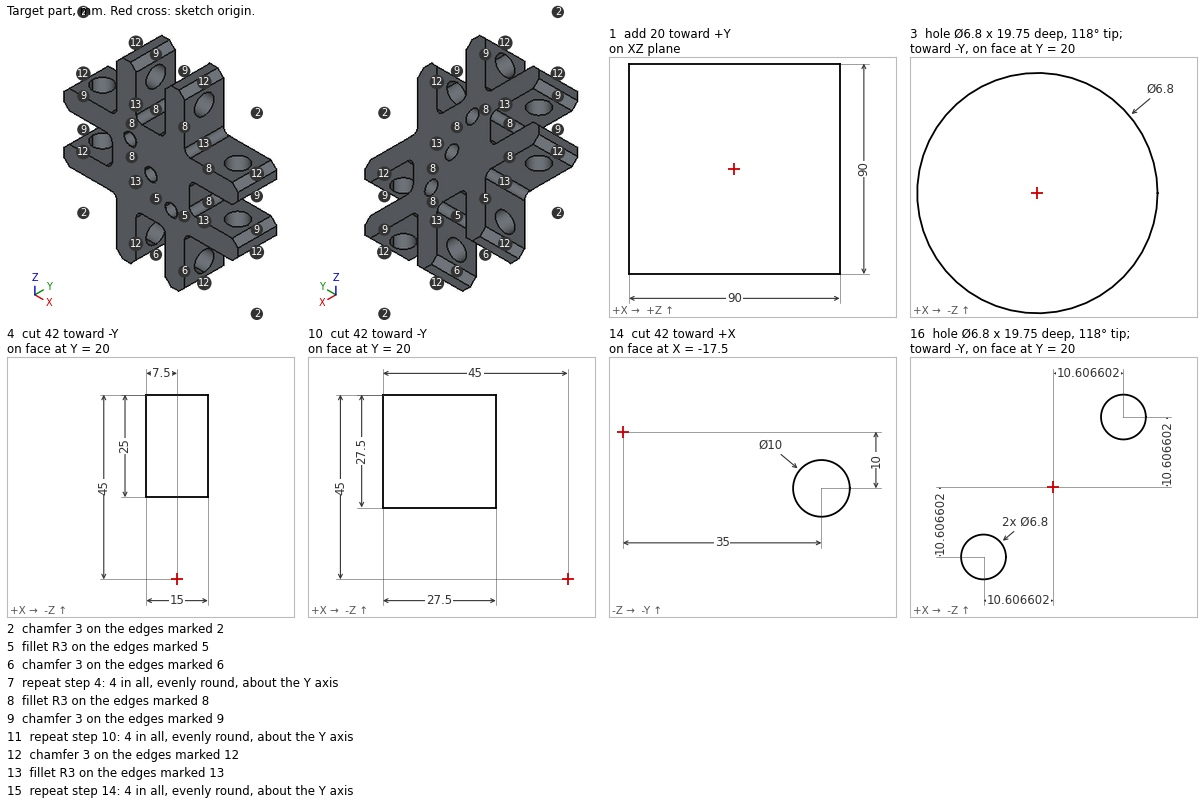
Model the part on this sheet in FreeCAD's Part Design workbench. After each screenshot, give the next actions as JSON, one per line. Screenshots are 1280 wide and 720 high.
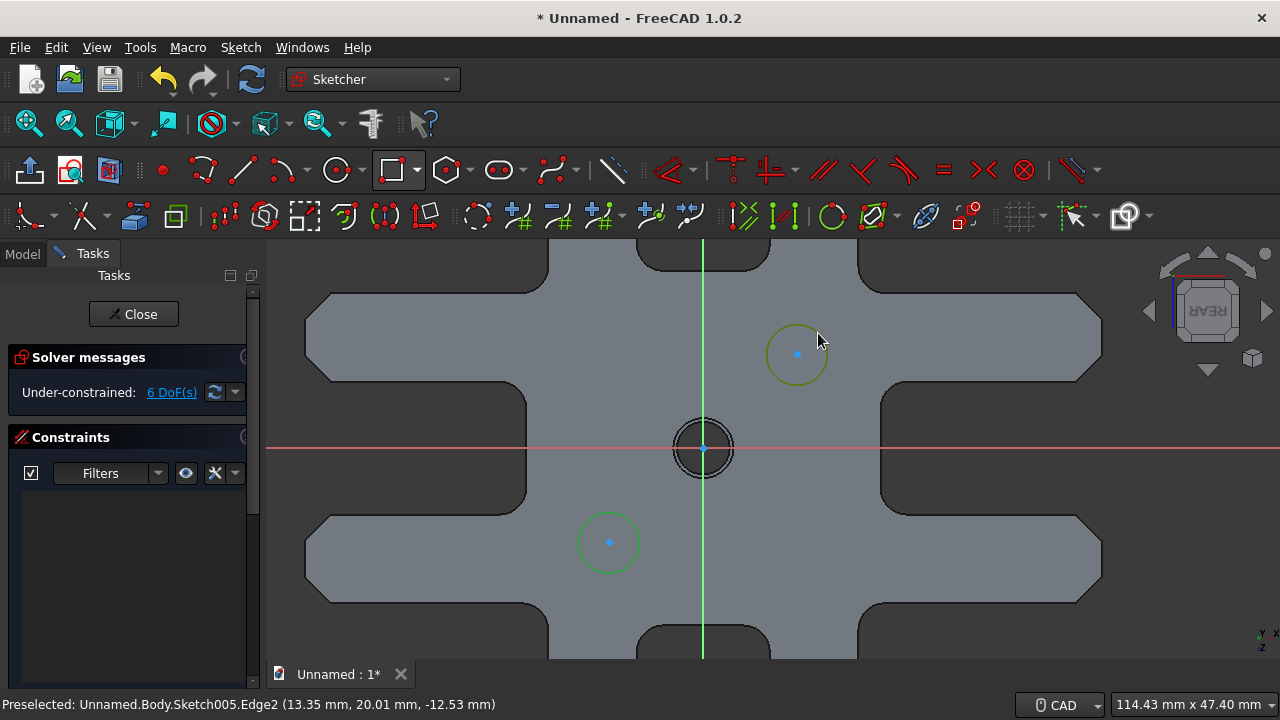
{"action": "left_click", "coordinate": [944, 170]}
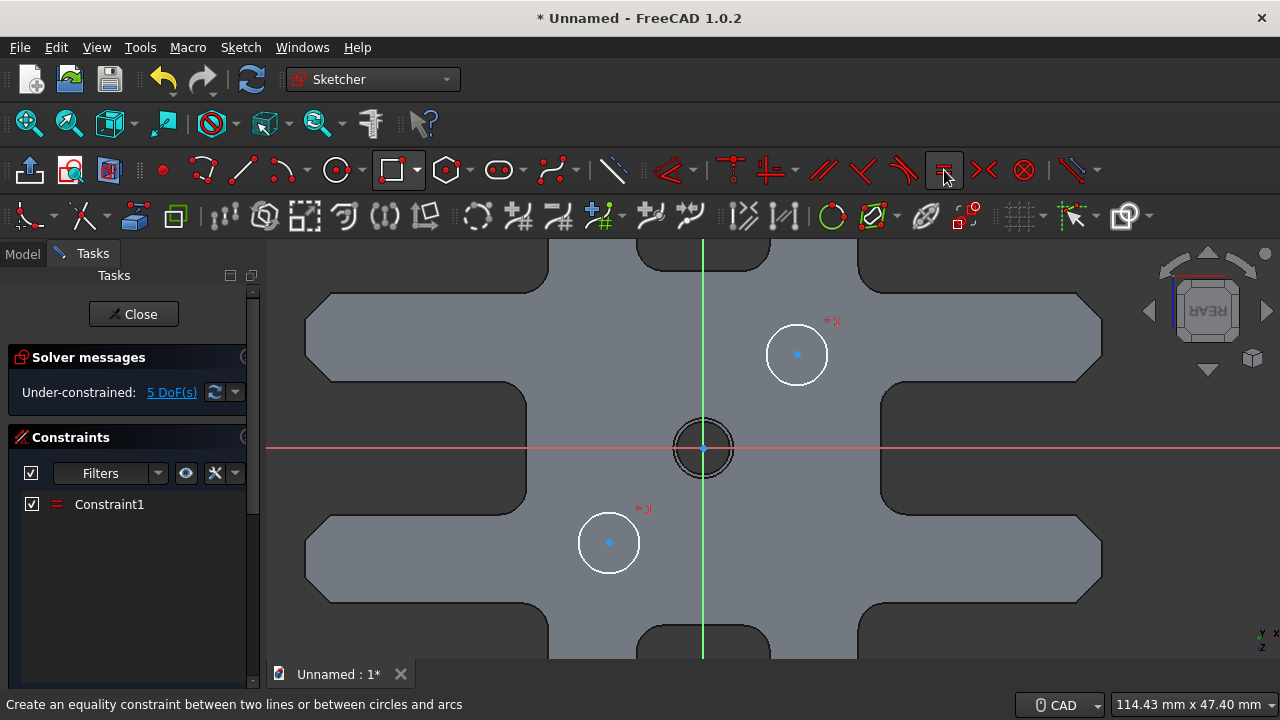
{"action": "left_click", "coordinate": [668, 170]}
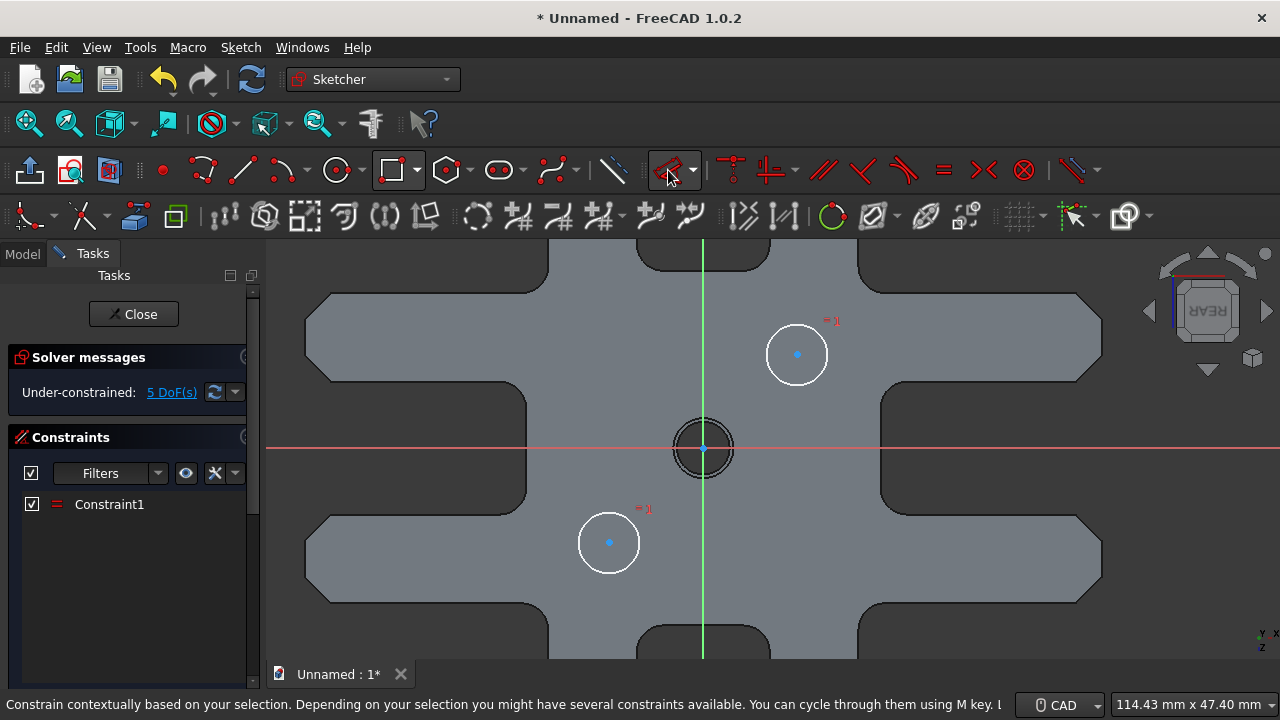
{"action": "left_click", "coordinate": [630, 521]}
{"action": "left_click", "coordinate": [652, 498]}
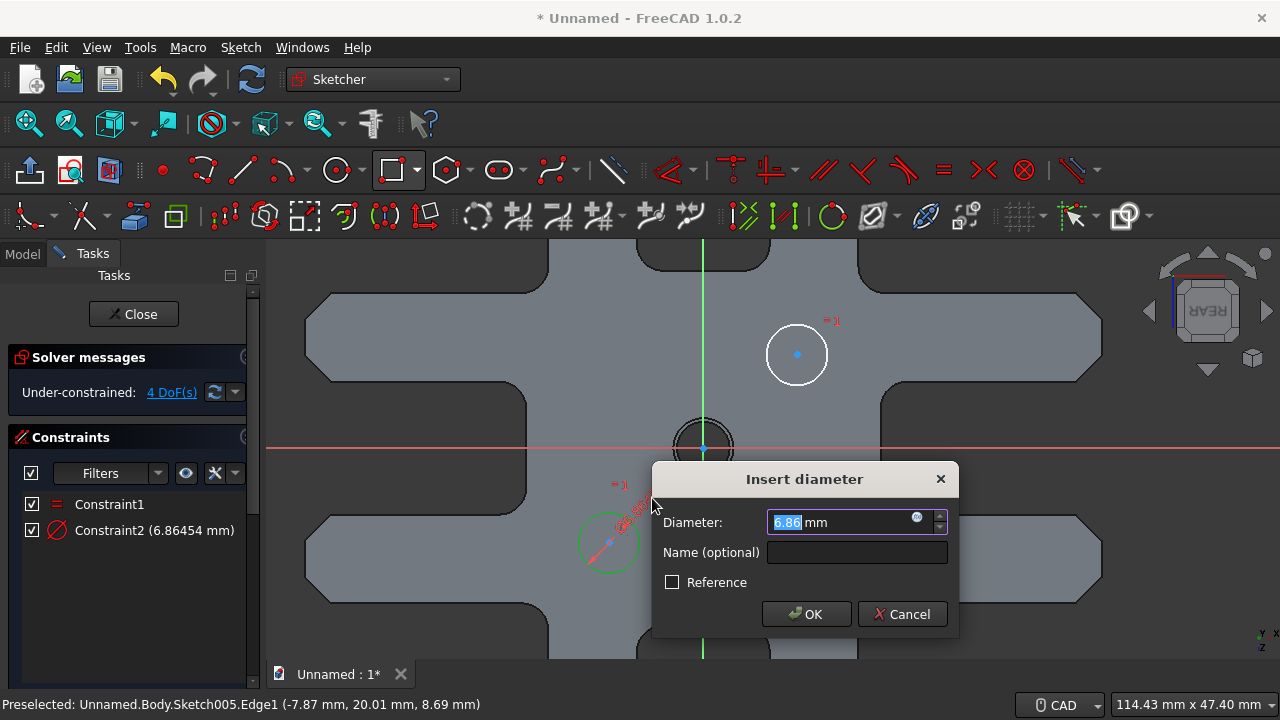
{"action": "type", "text": "6.8"}
{"action": "key", "text": "Return"}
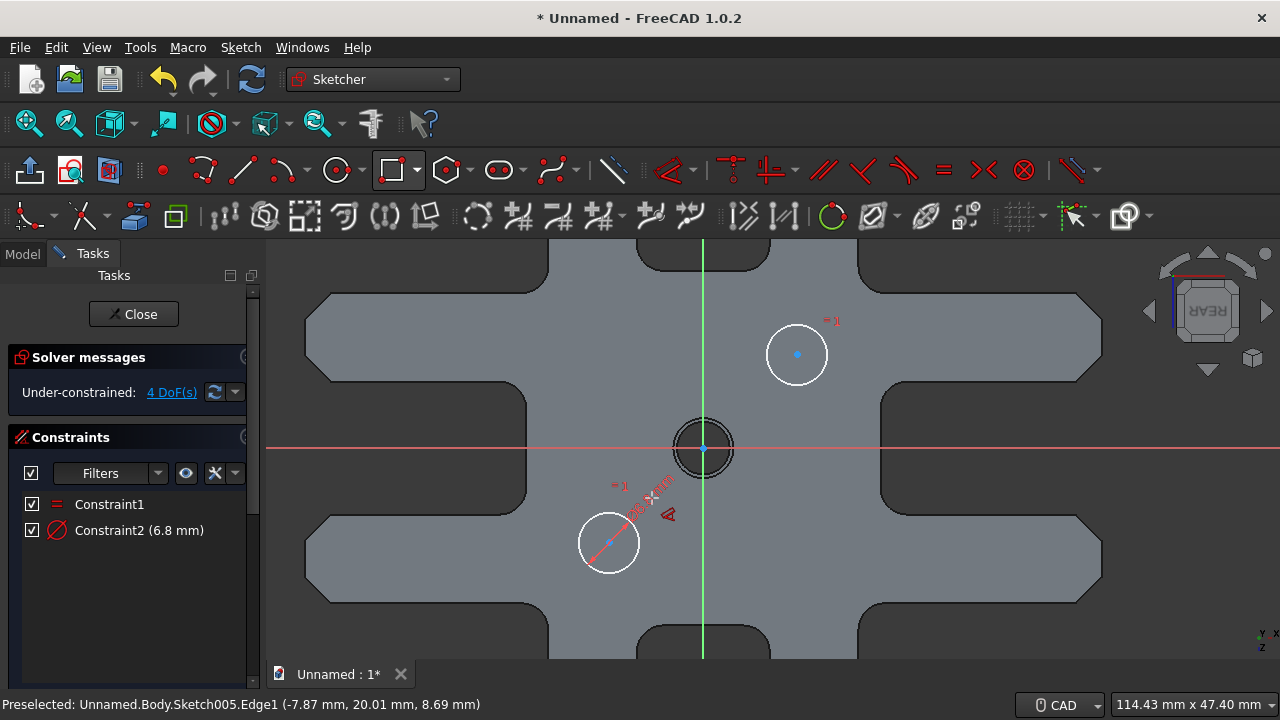
{"action": "left_click", "coordinate": [609, 543]}
{"action": "left_click", "coordinate": [656, 577]}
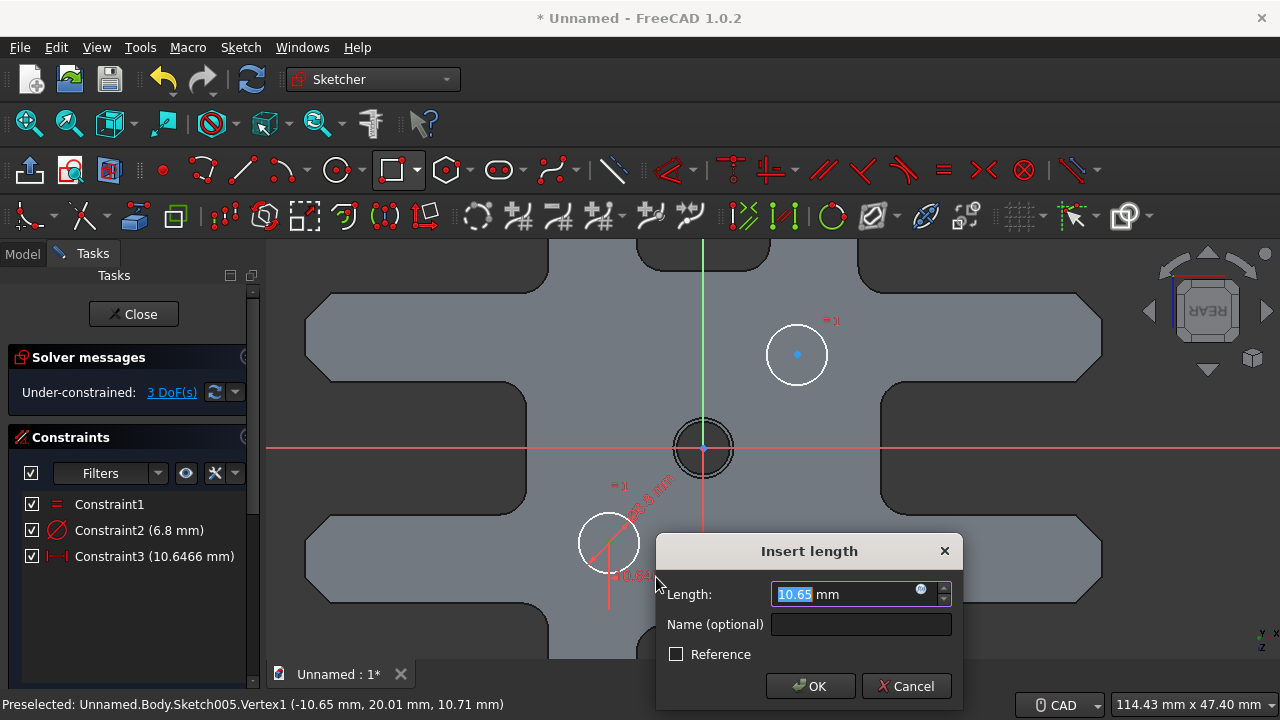
{"action": "type", "text": "10.606602"}
{"action": "key", "text": "Return"}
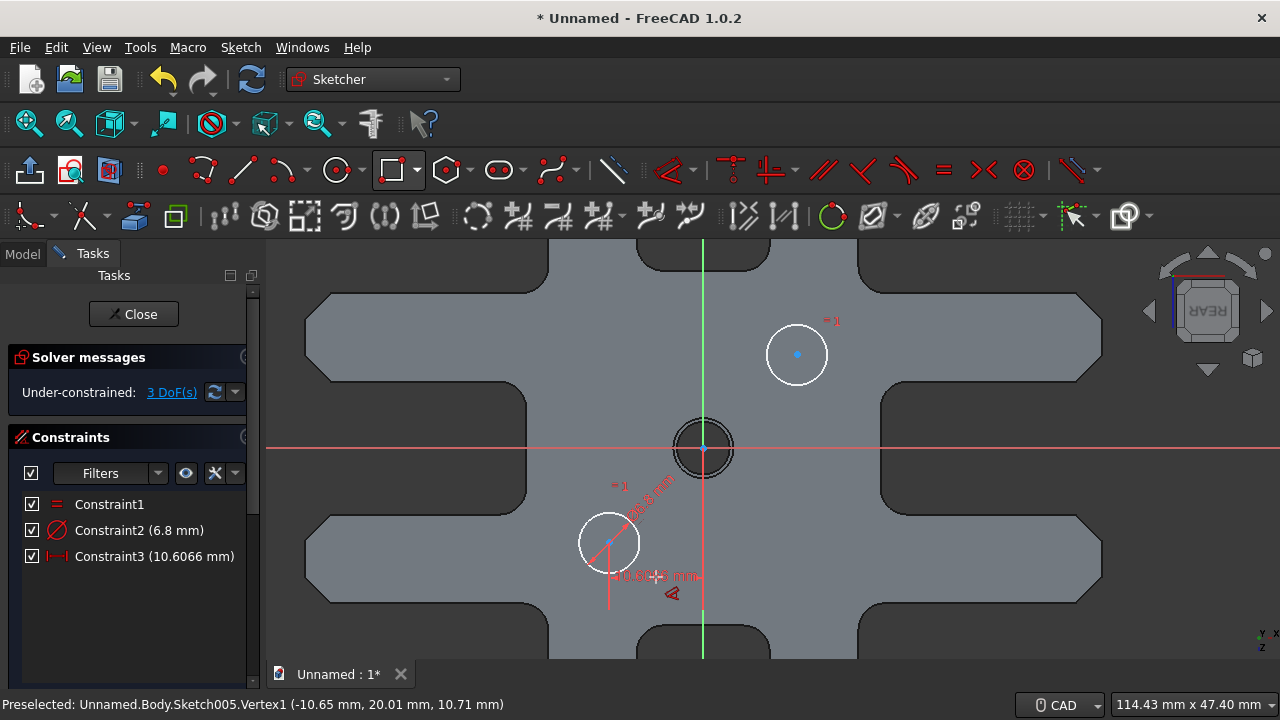
{"action": "left_click", "coordinate": [609, 543]}
{"action": "left_click", "coordinate": [575, 496]}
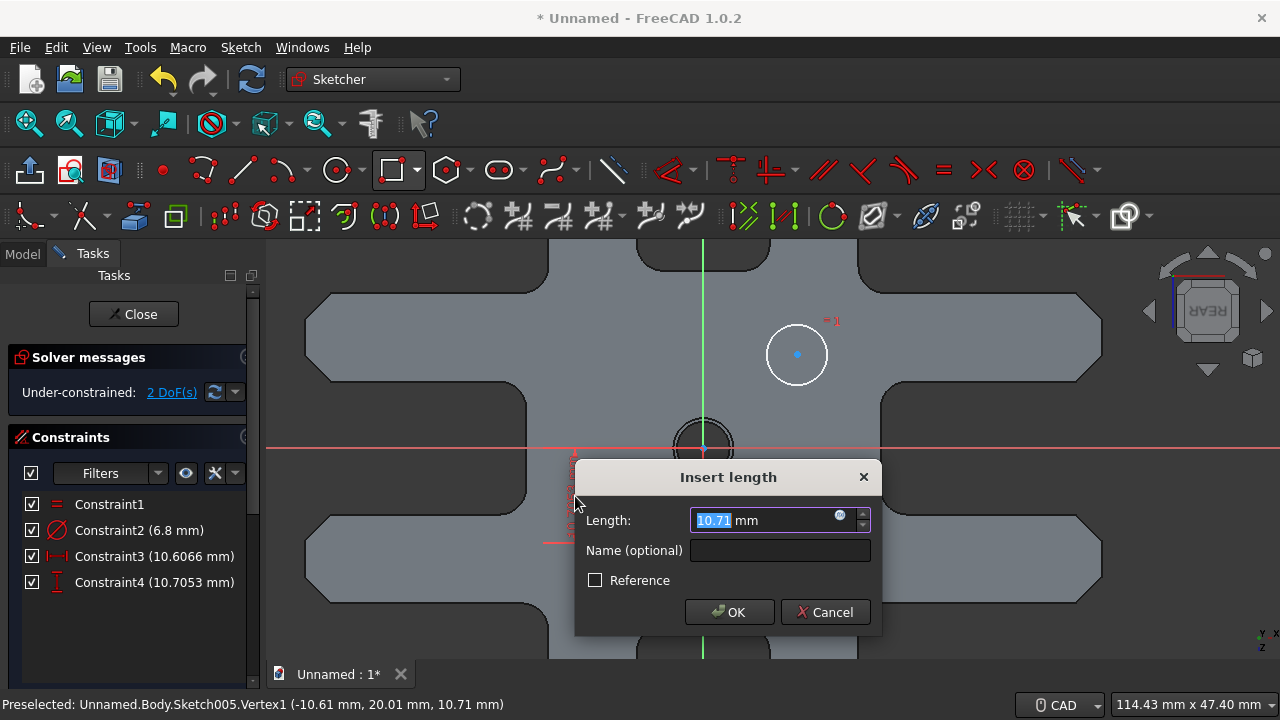
{"action": "type", "text": "10.606602"}
{"action": "key", "text": "Return"}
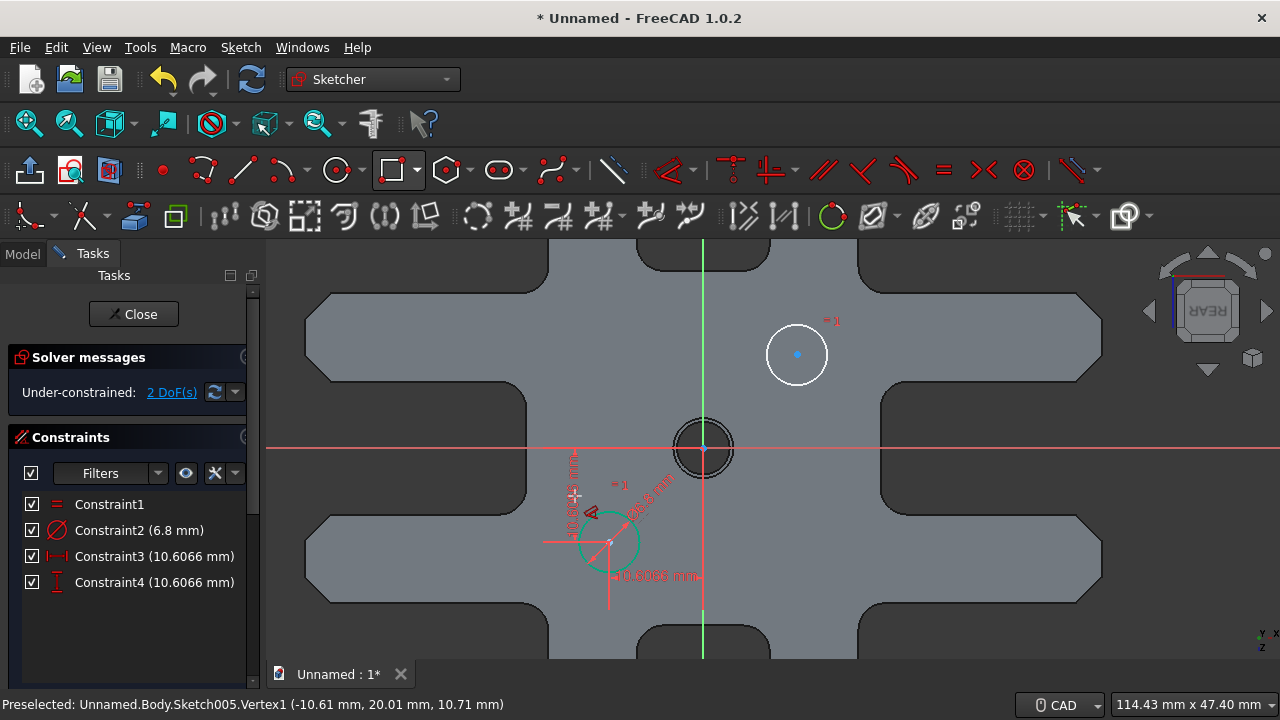
{"action": "left_click", "coordinate": [797, 355]}
{"action": "left_click", "coordinate": [750, 321]}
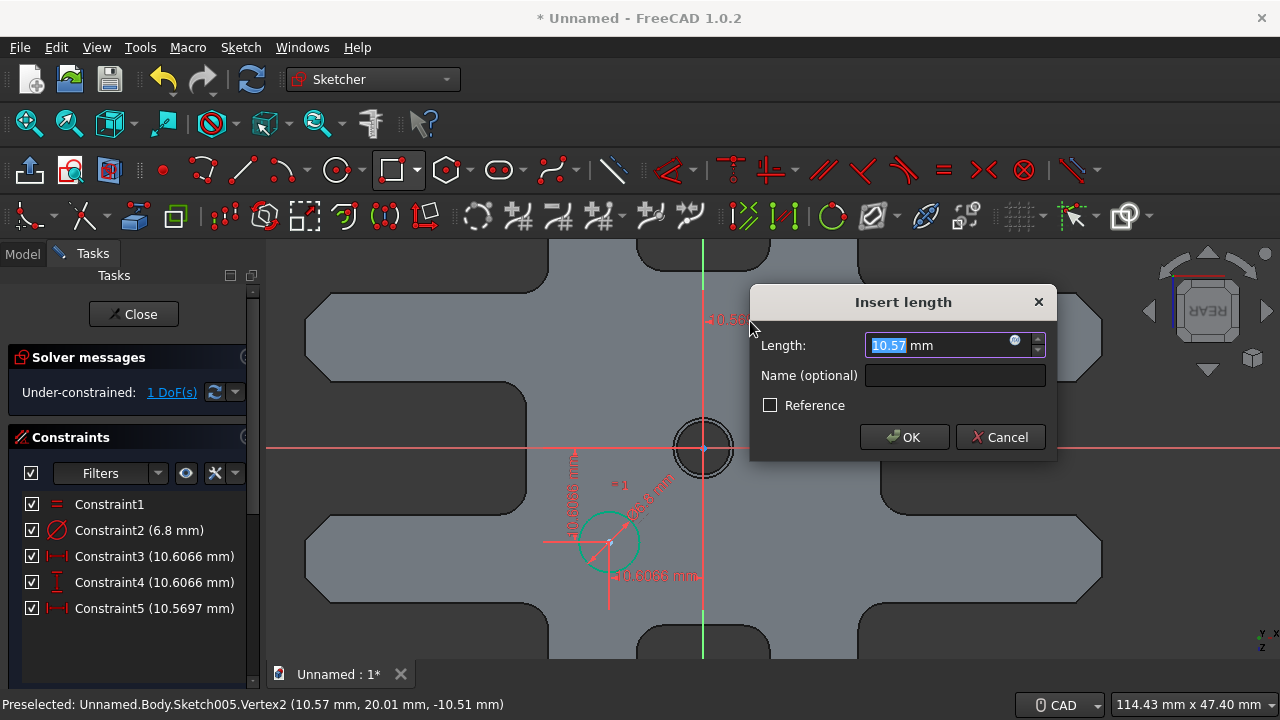
{"action": "type", "text": "10.606602"}
{"action": "key", "text": "Return"}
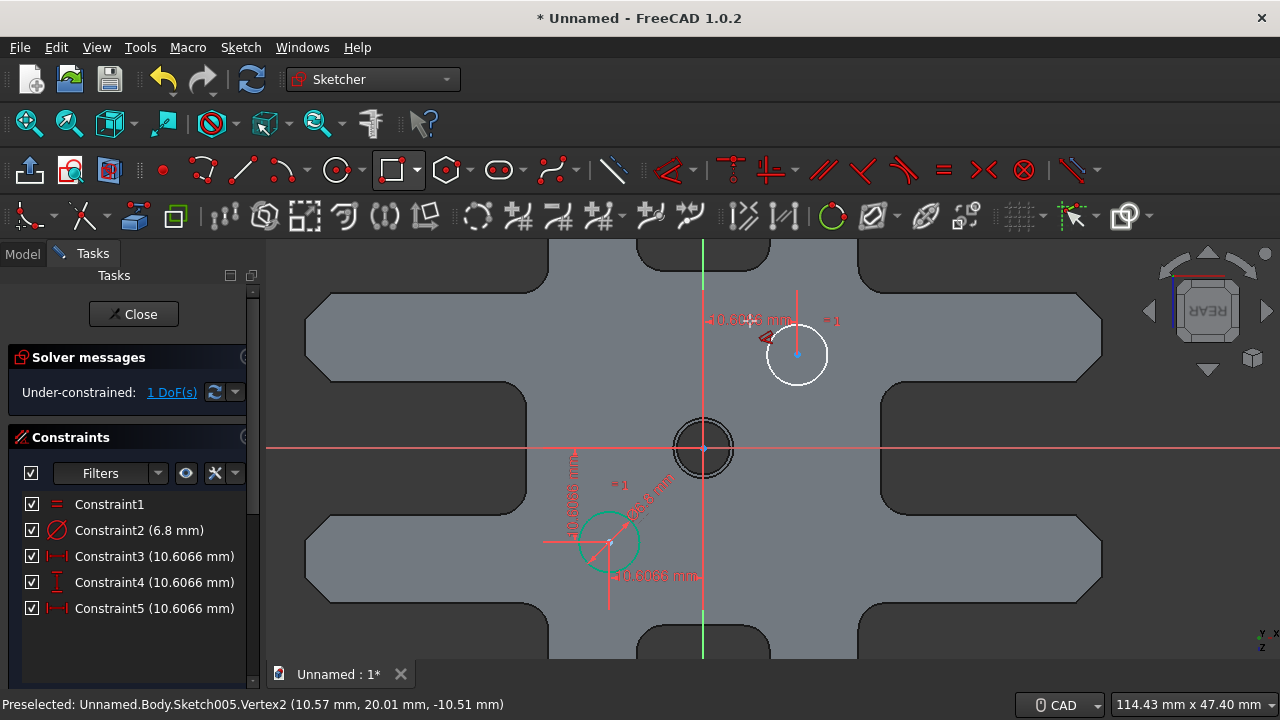
{"action": "left_click", "coordinate": [797, 355]}
{"action": "left_click", "coordinate": [831, 402]}